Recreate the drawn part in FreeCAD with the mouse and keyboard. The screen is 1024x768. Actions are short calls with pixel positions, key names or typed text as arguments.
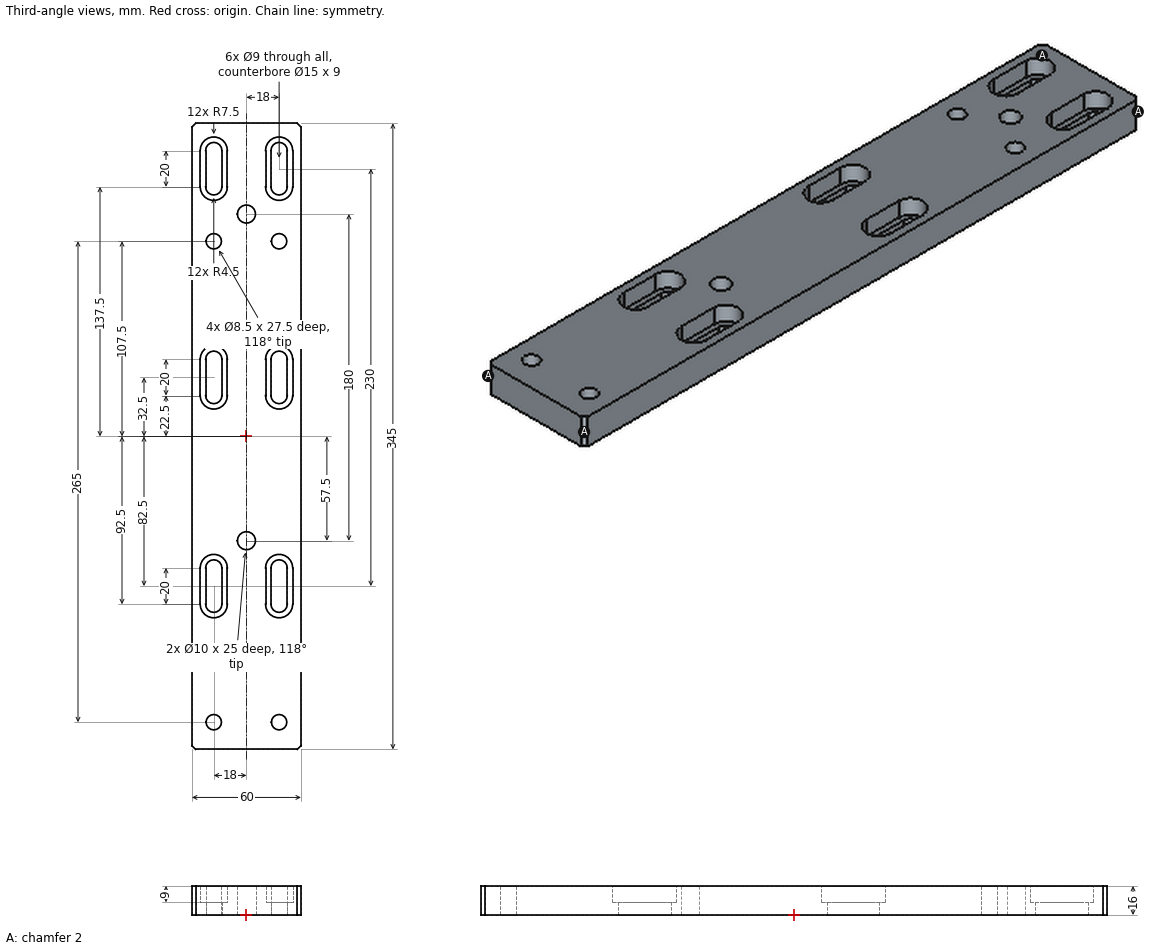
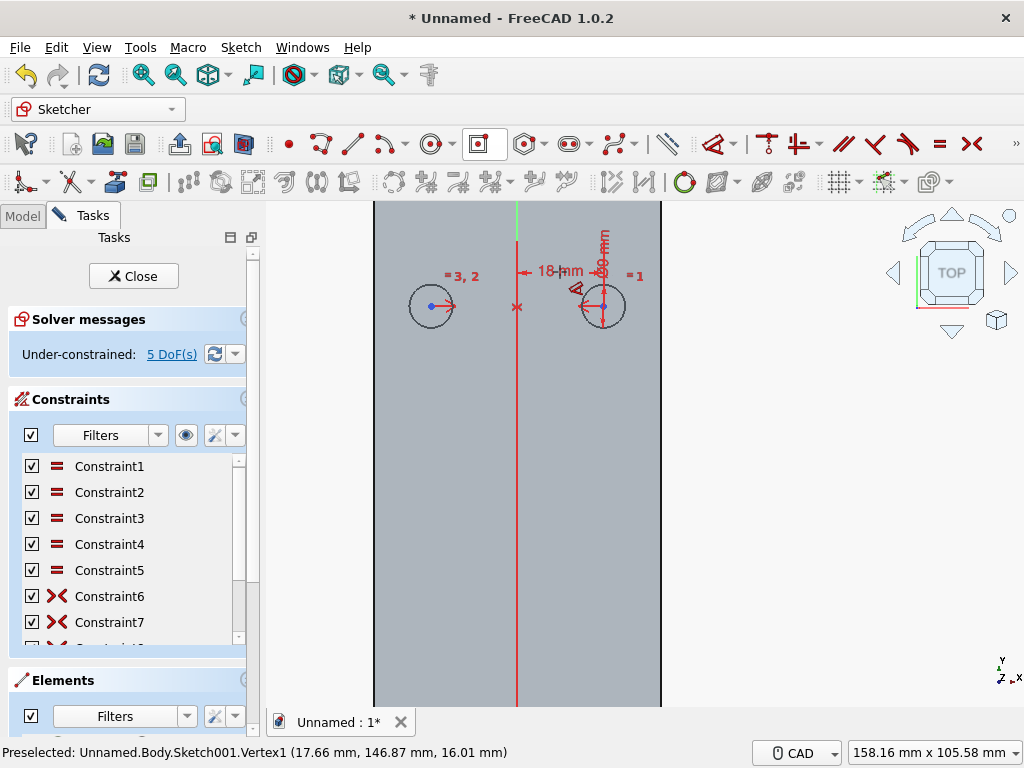
scroll(602, 281, down, 6)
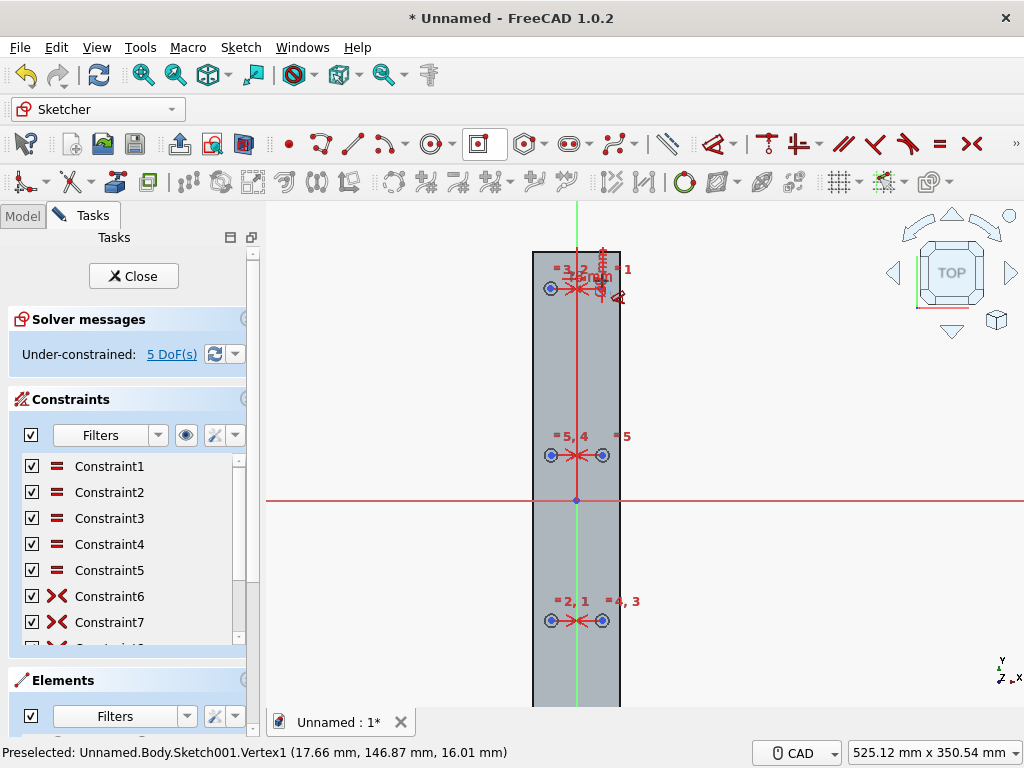
scroll(551, 621, up, 3)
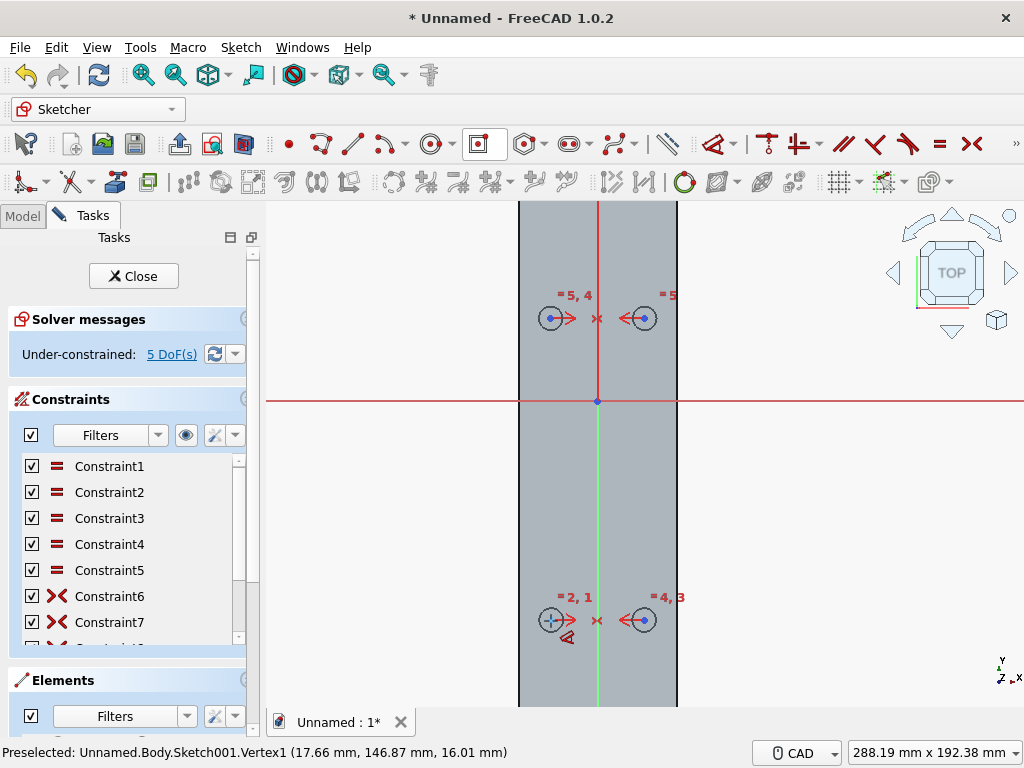
click(551, 620)
click(574, 654)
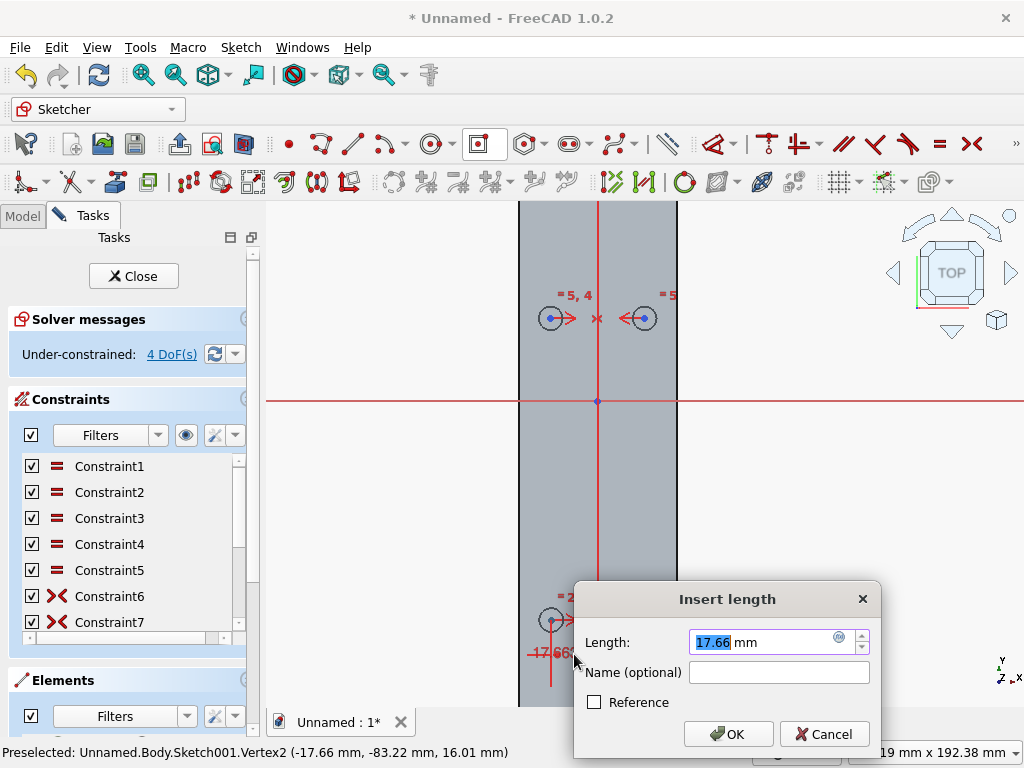
text(18)
key(Return)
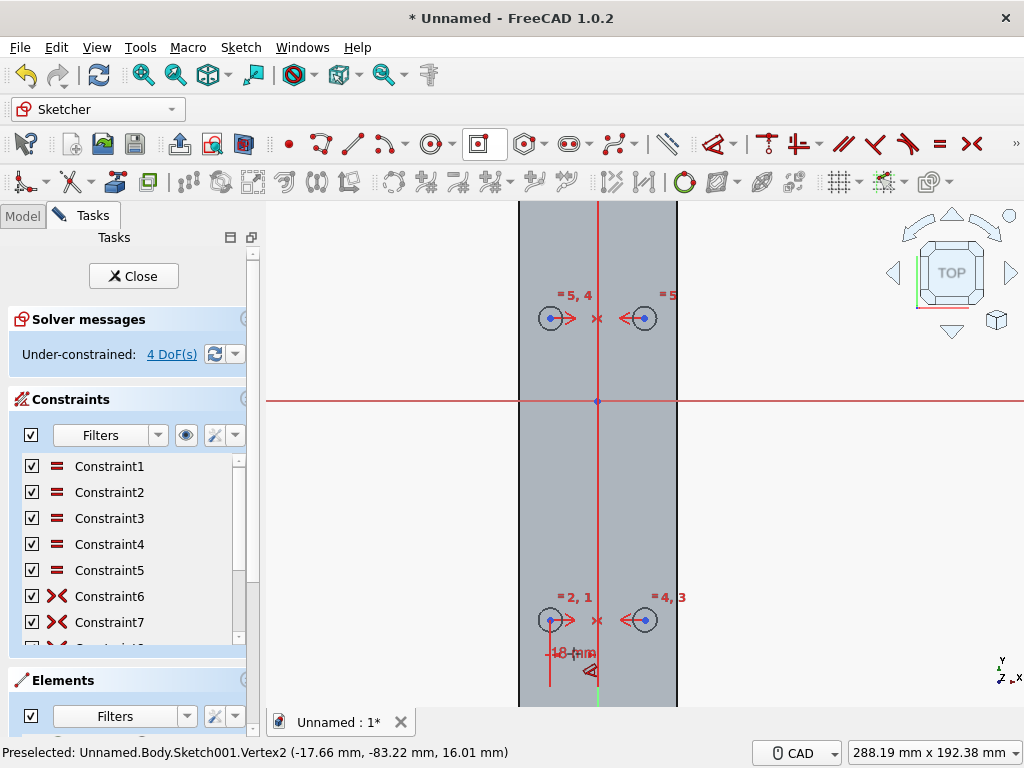
click(551, 318)
click(574, 435)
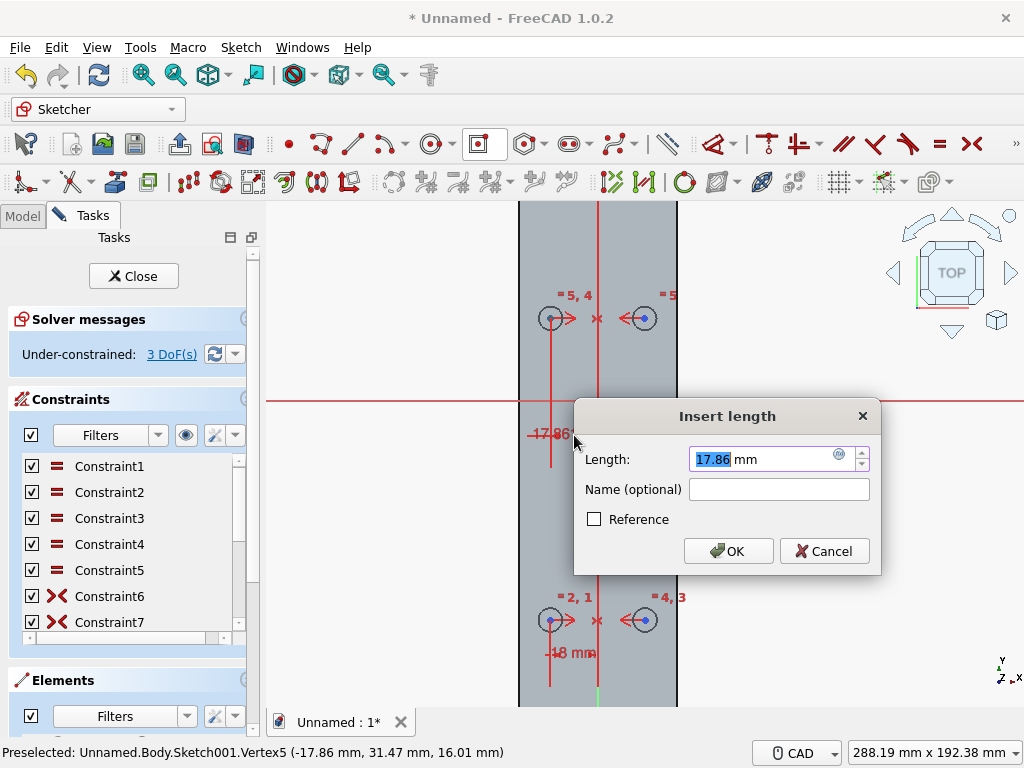
text(18)
key(Return)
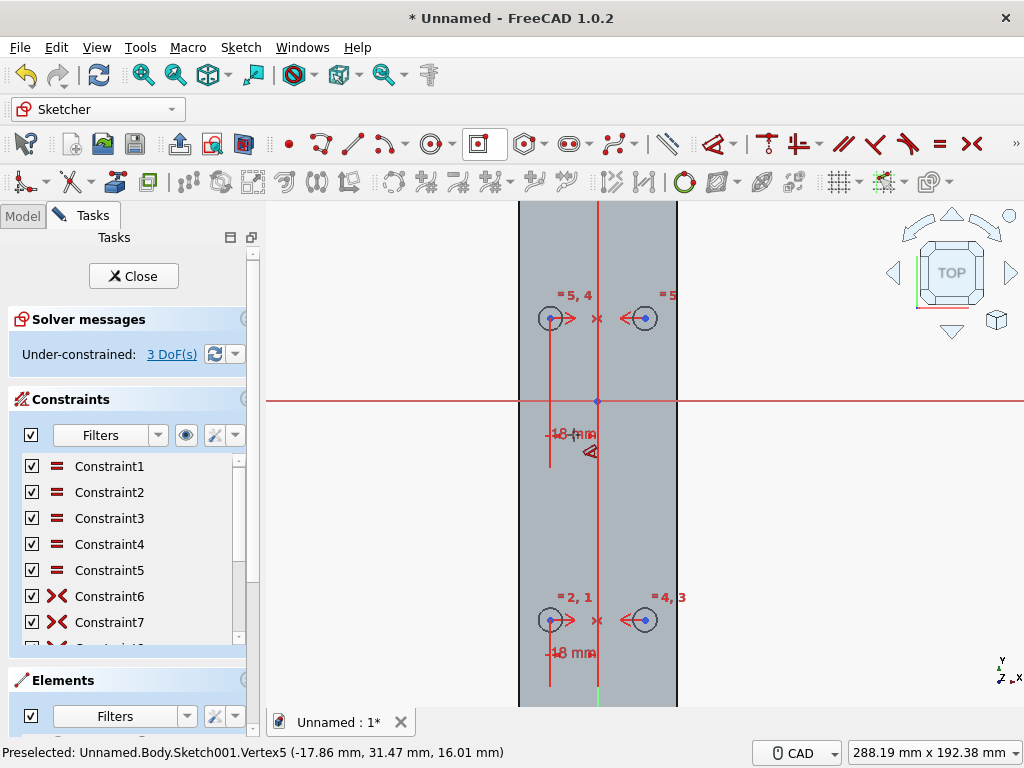
click(550, 620)
click(516, 511)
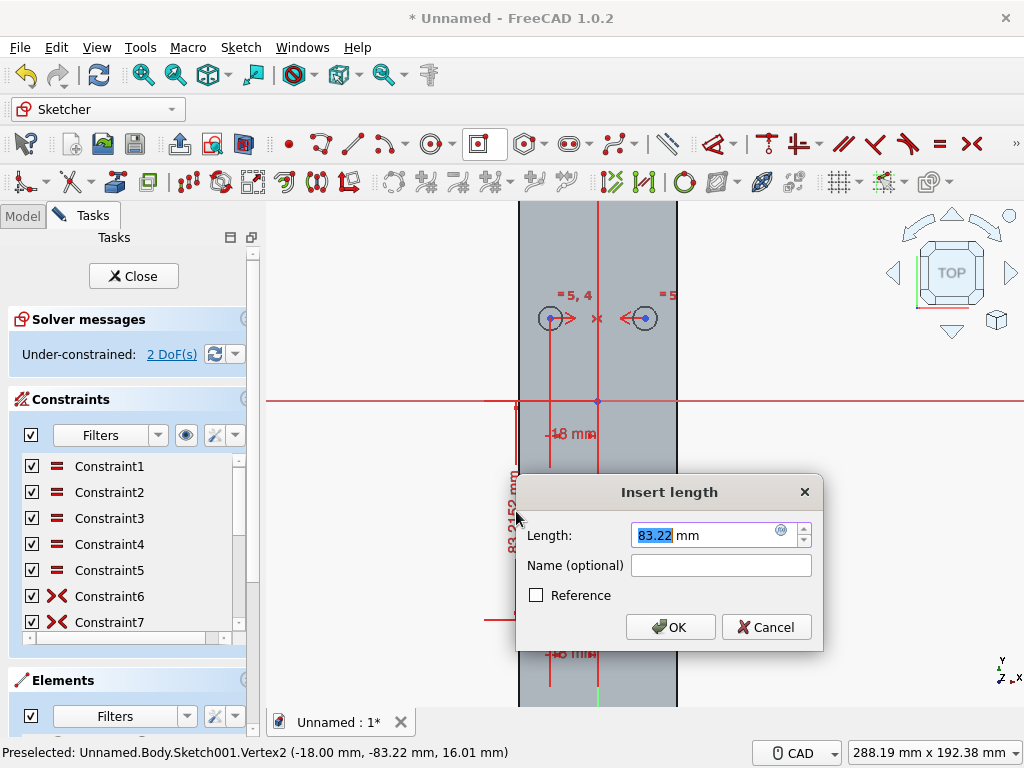
text(82.5)
key(Return)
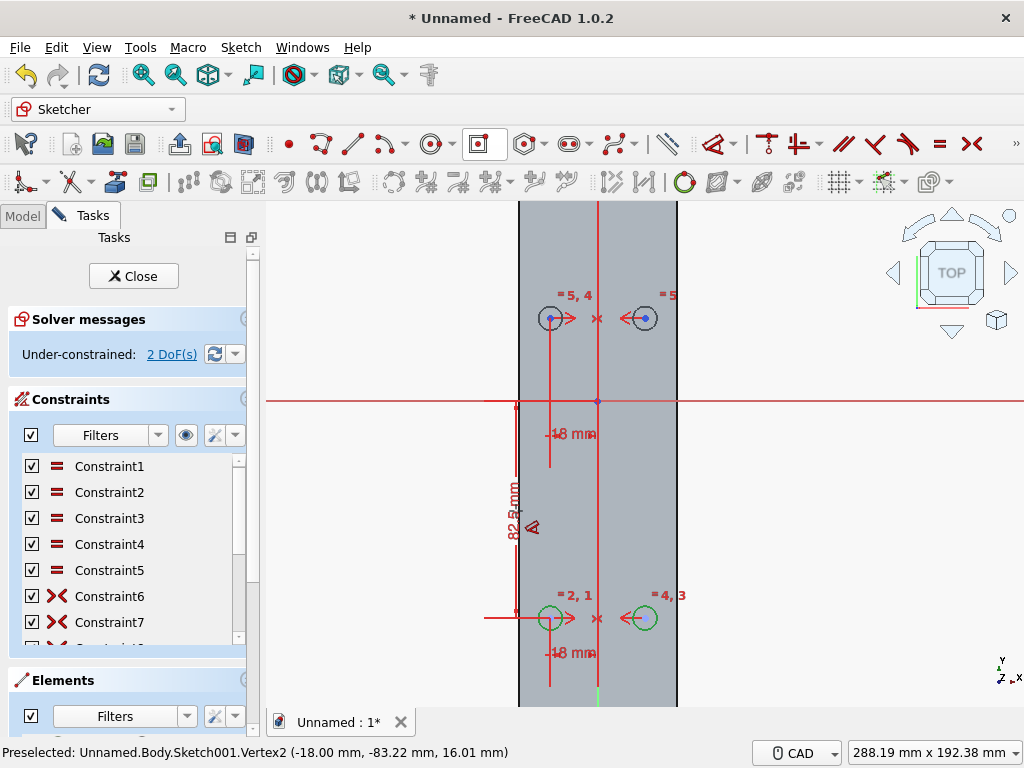
click(550, 318)
click(516, 360)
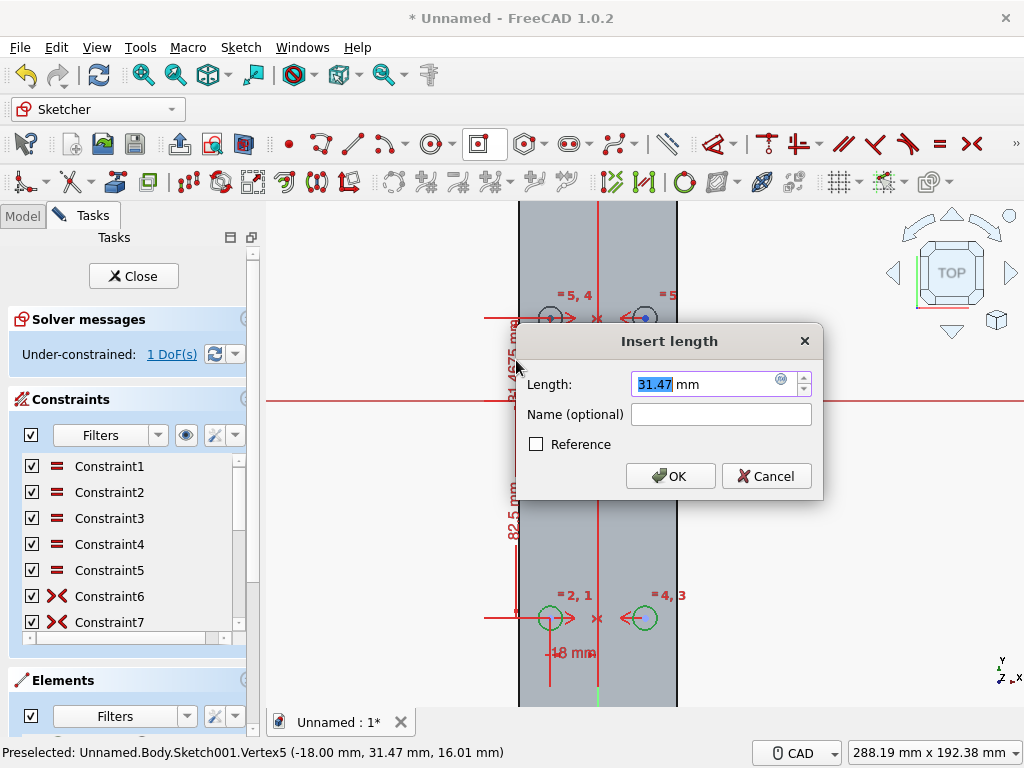
text(32.5)
key(Return)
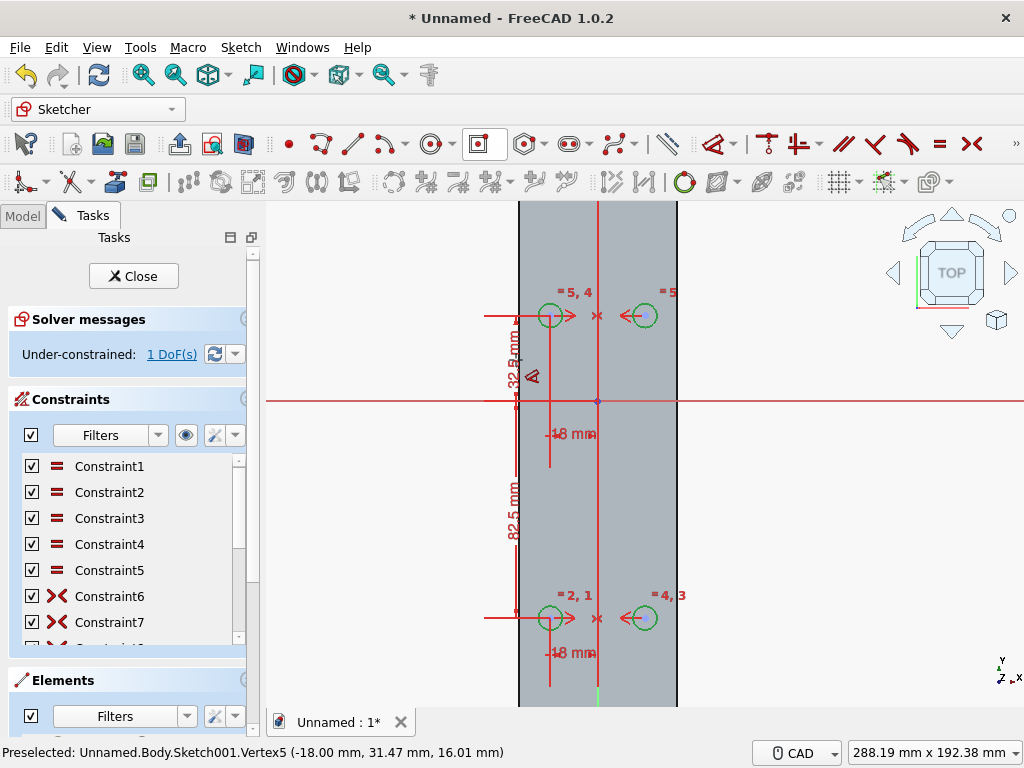
scroll(551, 622, down, 3)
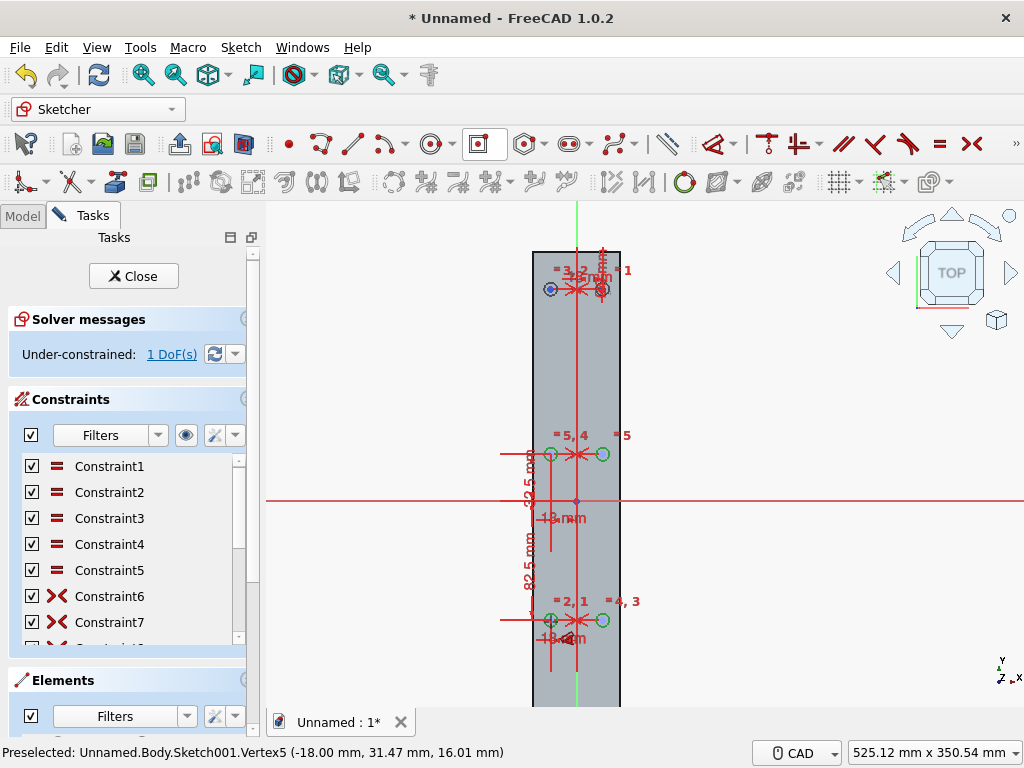
click(603, 289)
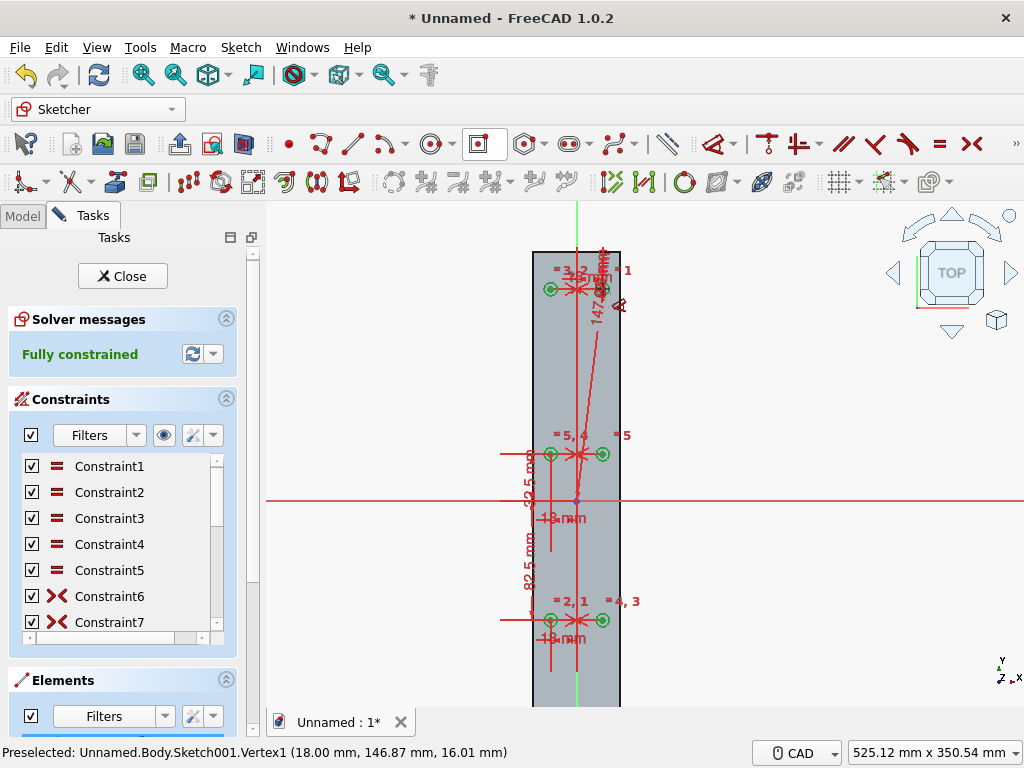
click(551, 620)
click(637, 455)